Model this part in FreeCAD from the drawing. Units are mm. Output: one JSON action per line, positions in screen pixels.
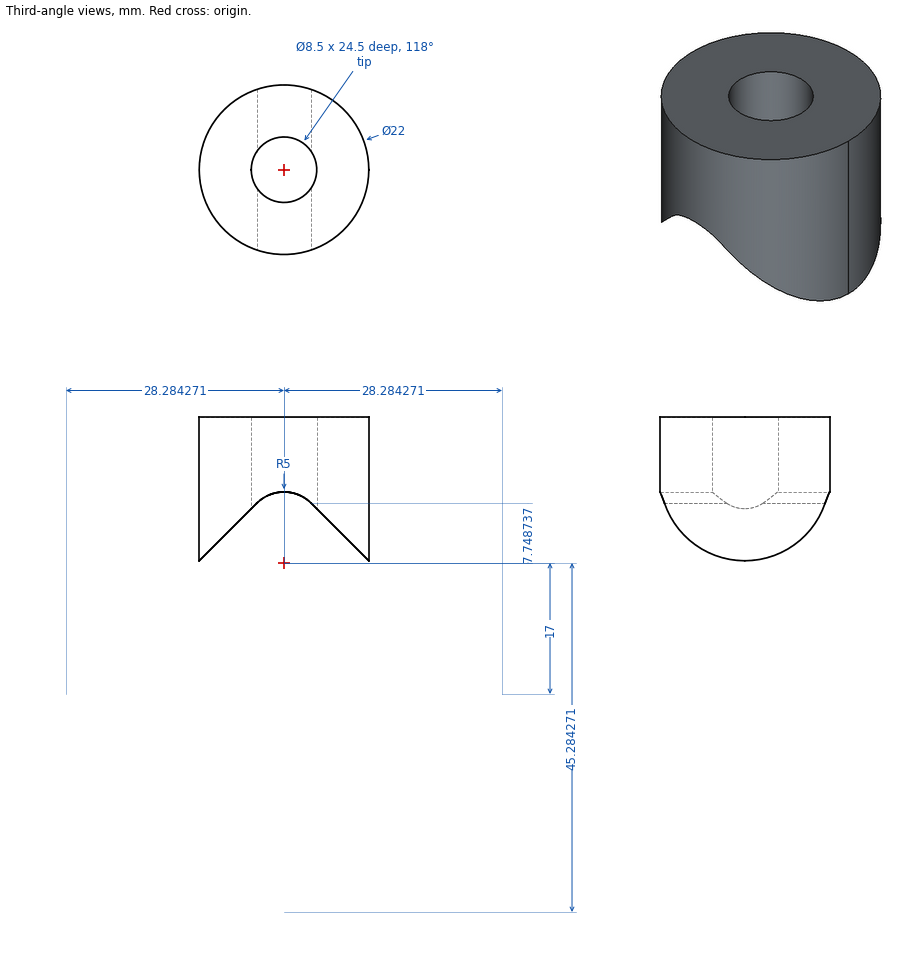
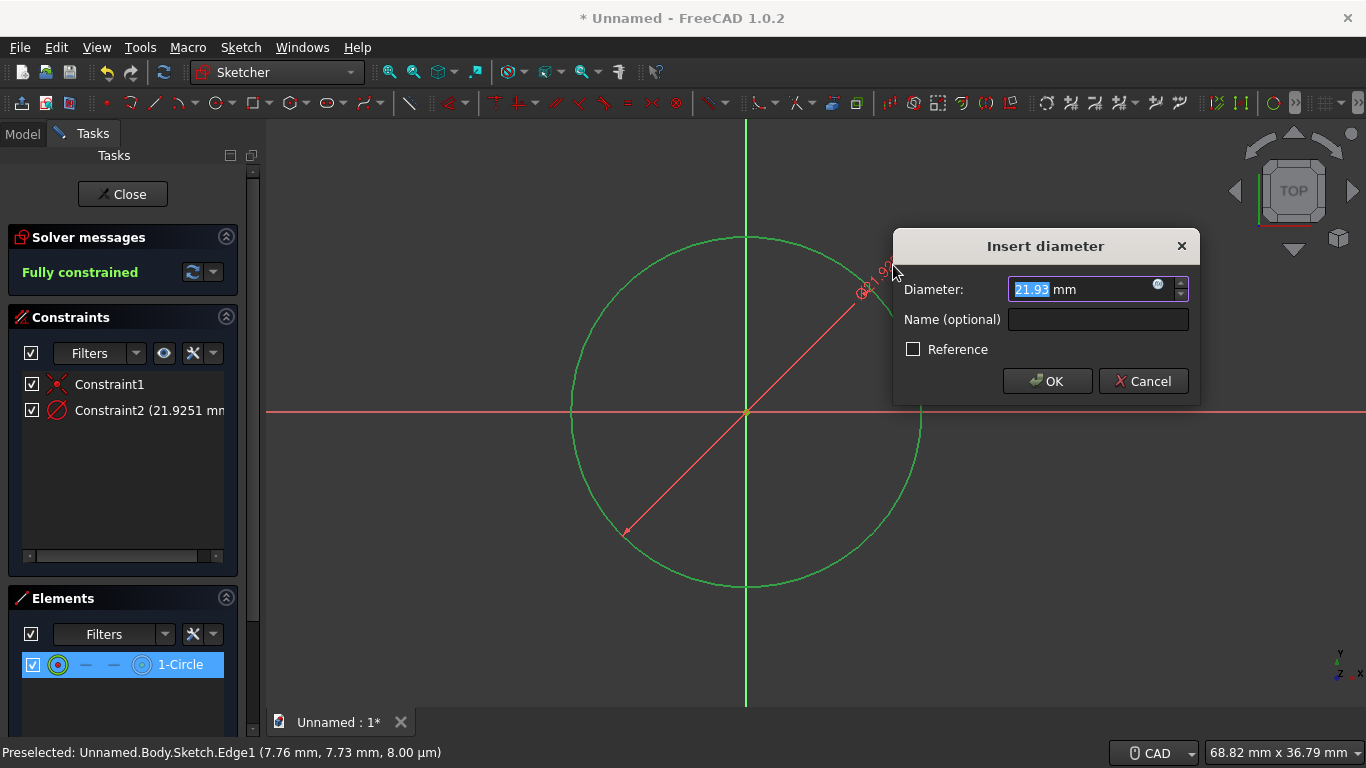
{"action": "type", "text": "22"}
{"action": "key", "text": "Return"}
{"action": "key", "text": "Escape"}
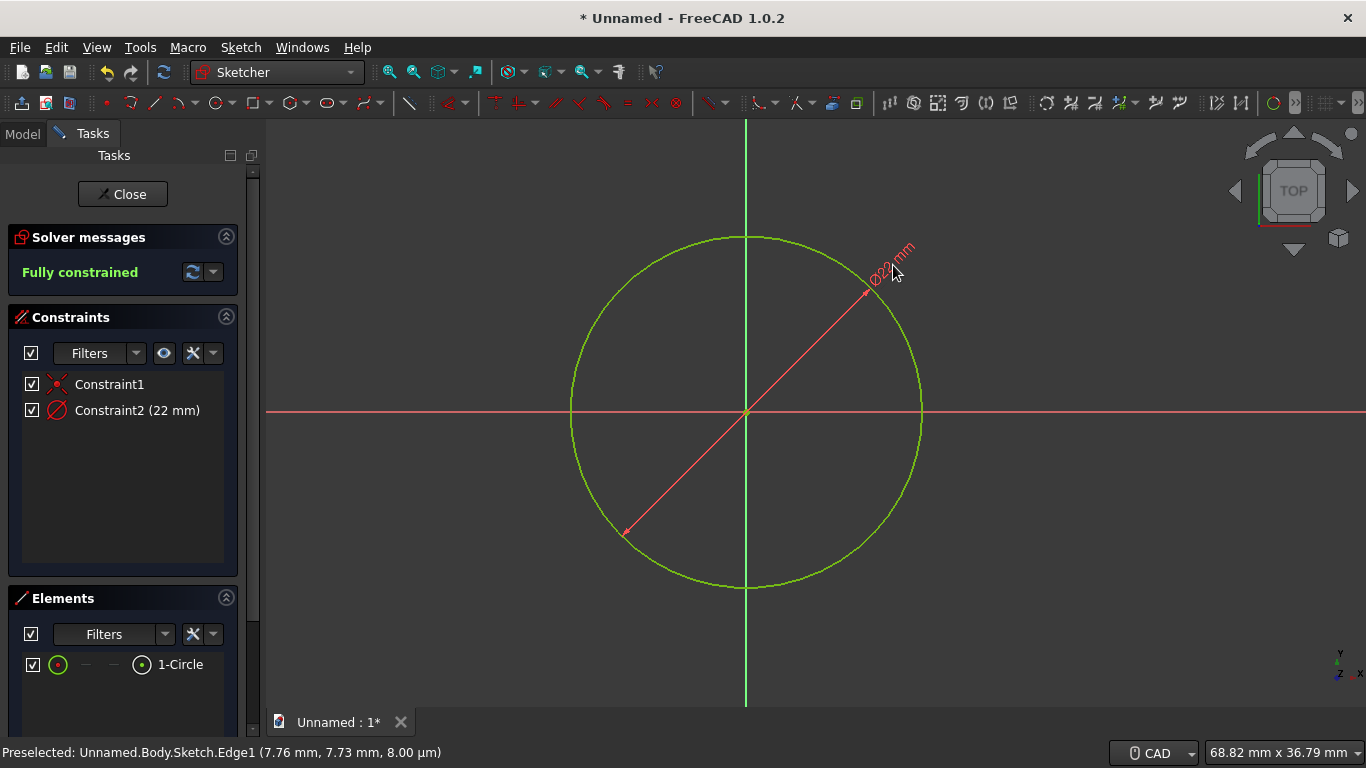
{"action": "left_click", "coordinate": [123, 194]}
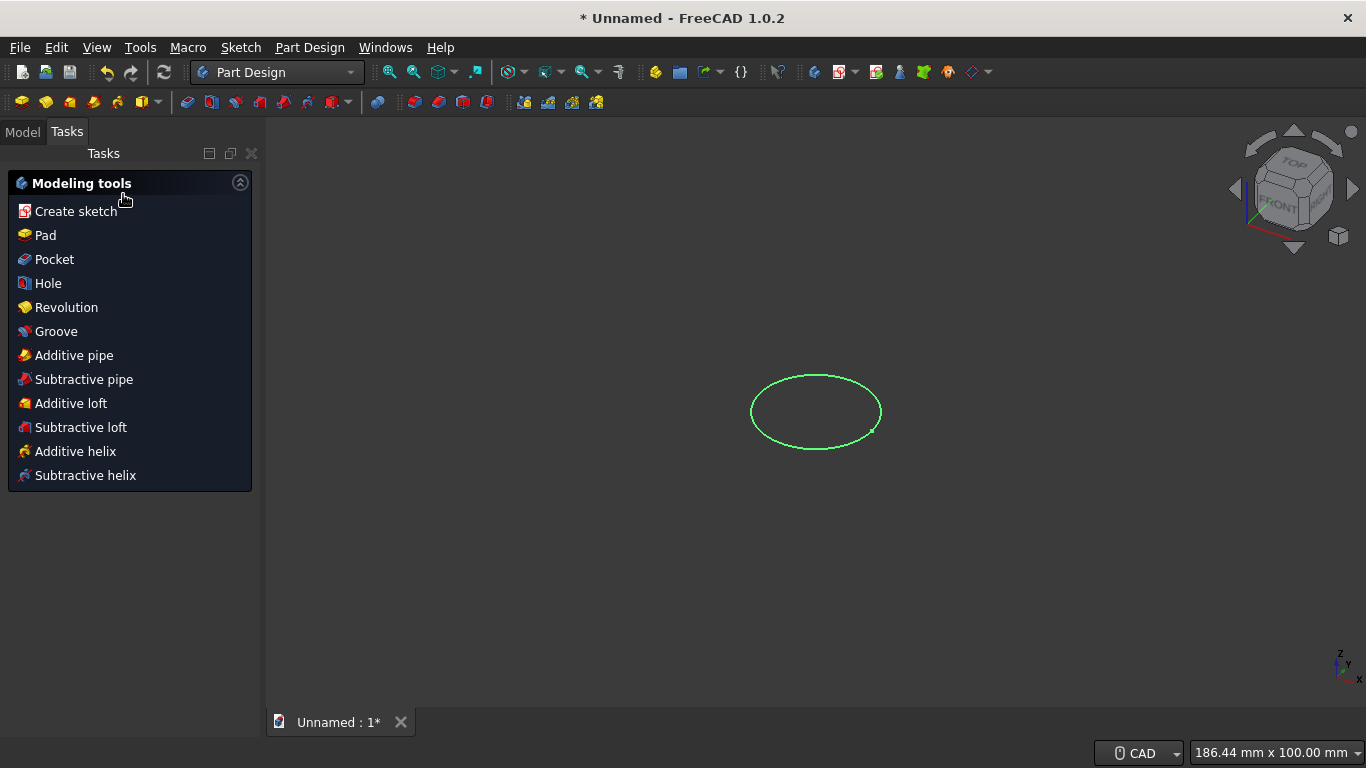
{"action": "left_click", "coordinate": [22, 102]}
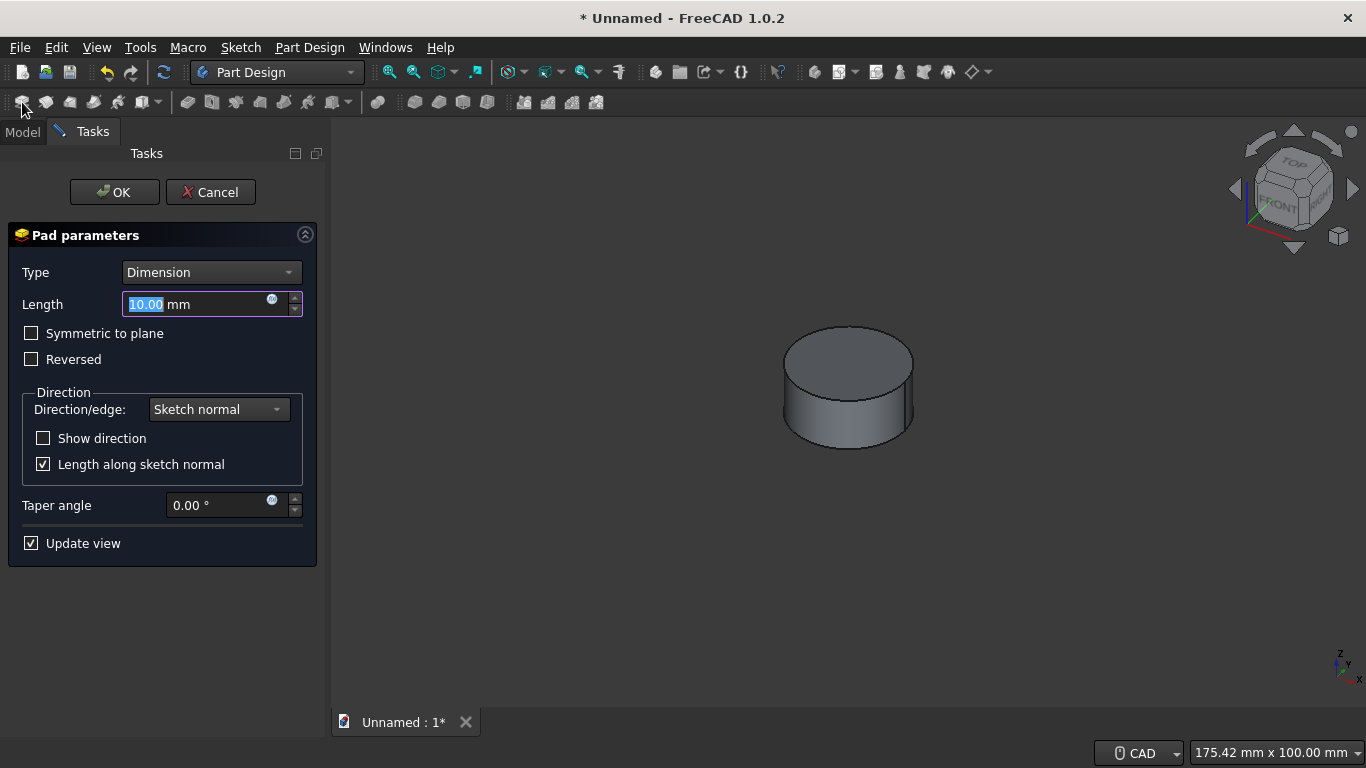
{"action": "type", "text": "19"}
{"action": "key", "text": "Tab"}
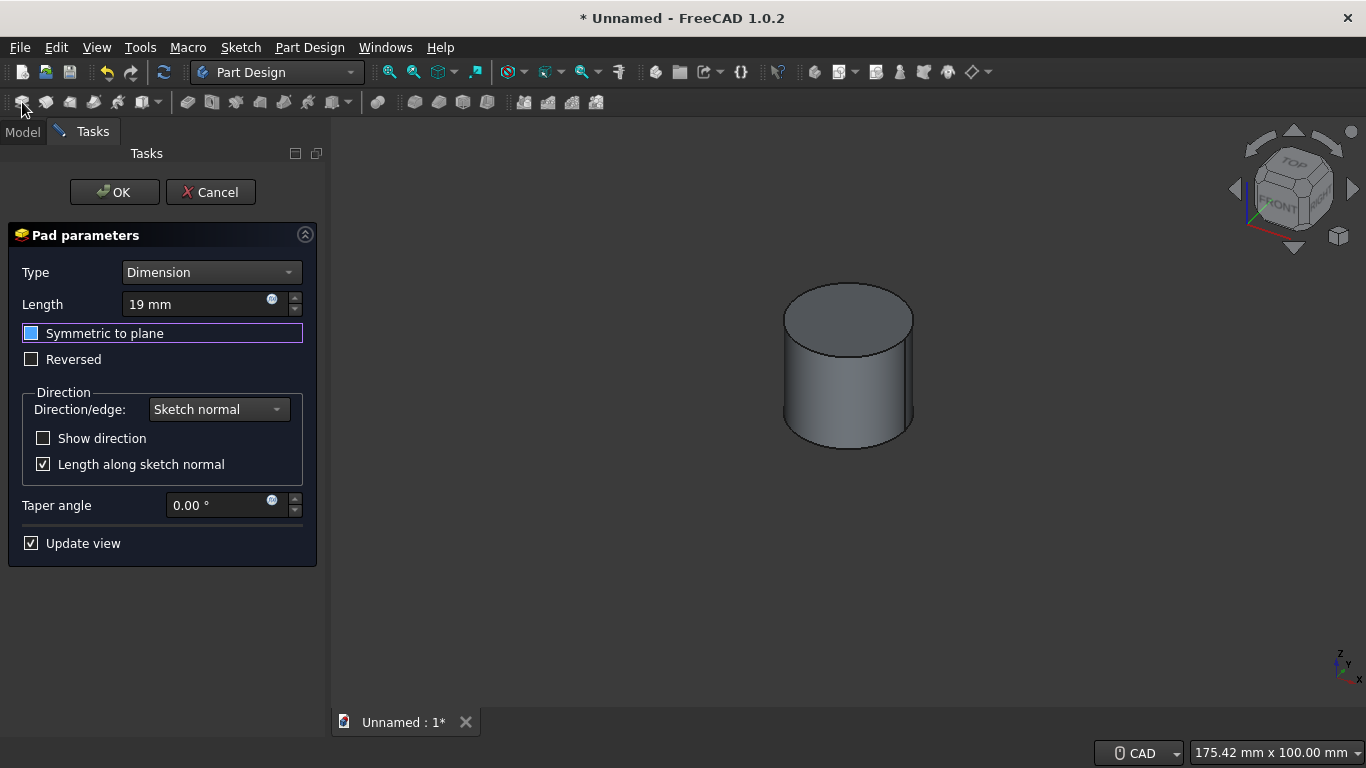
{"action": "left_click", "coordinate": [115, 192]}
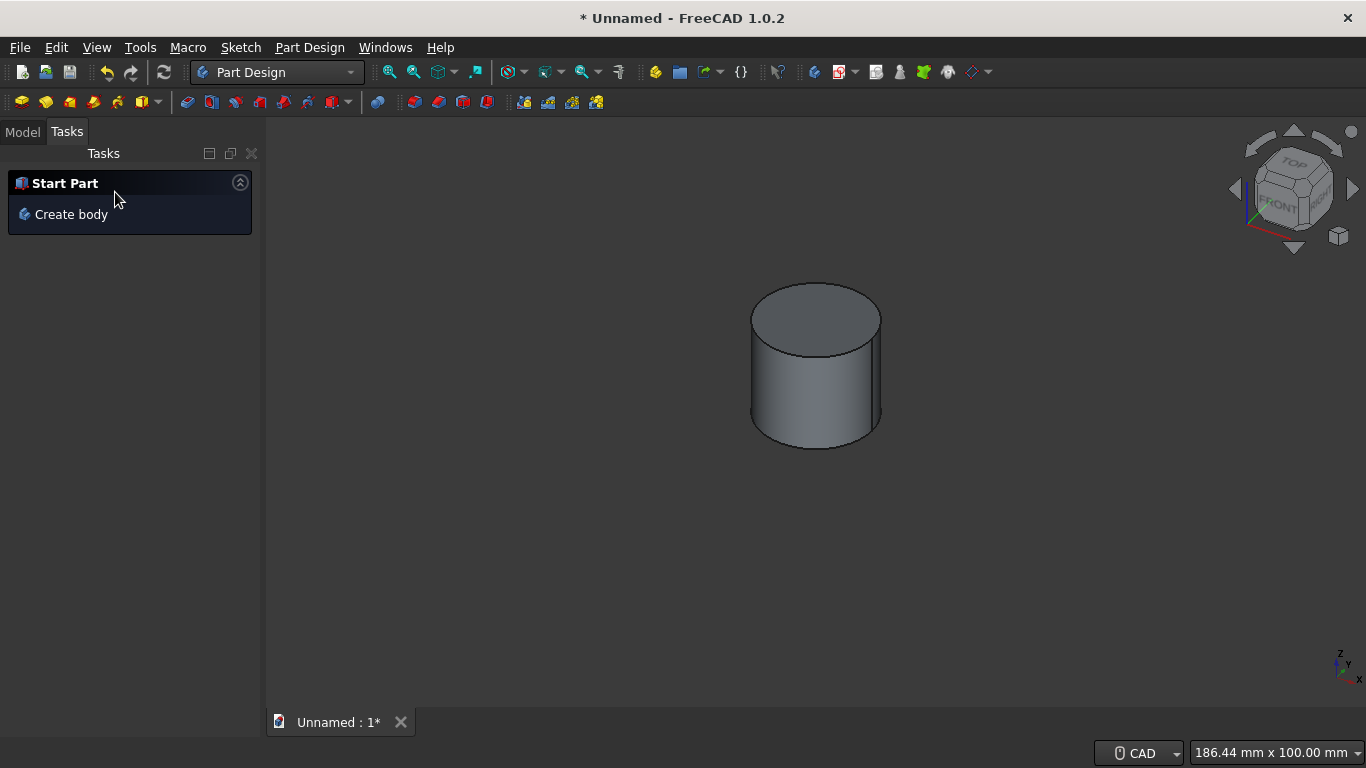
{"action": "key", "text": "v f"}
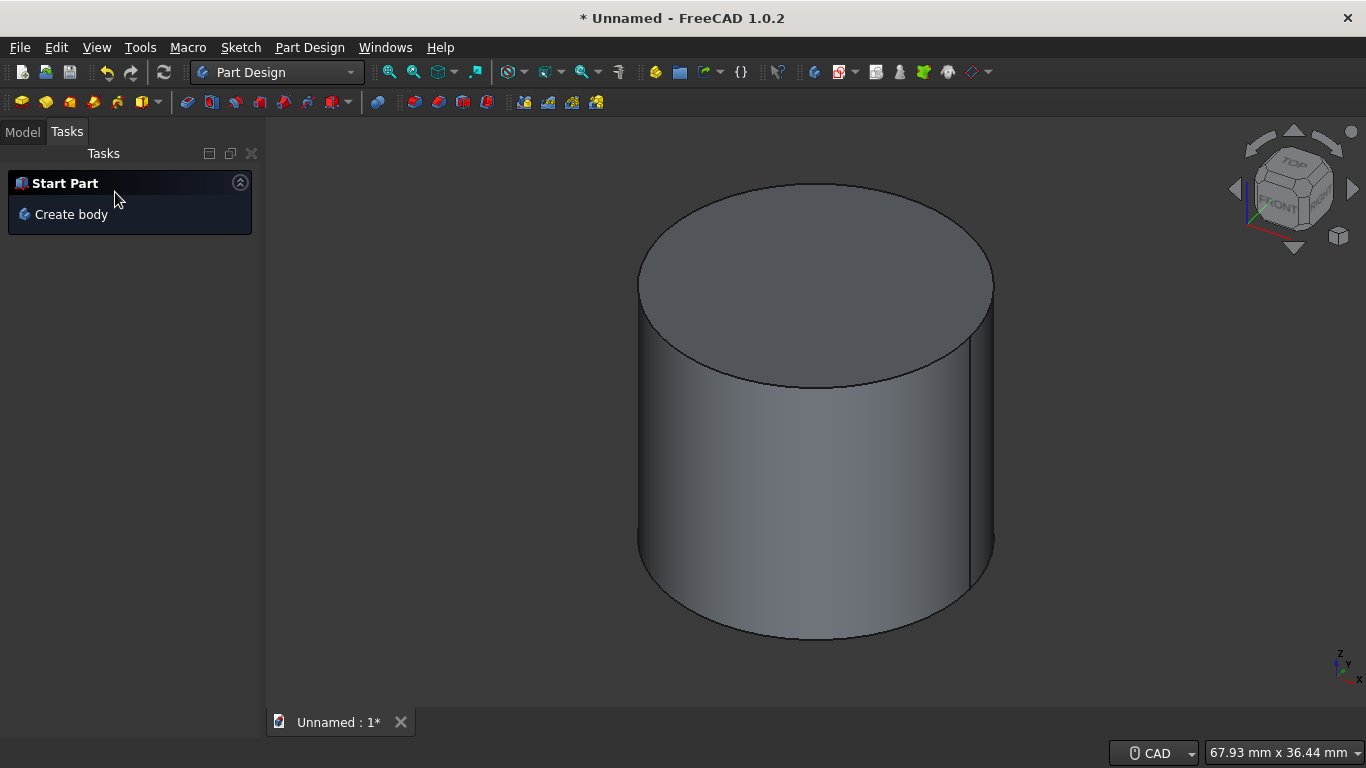
{"action": "left_click", "coordinate": [816, 285]}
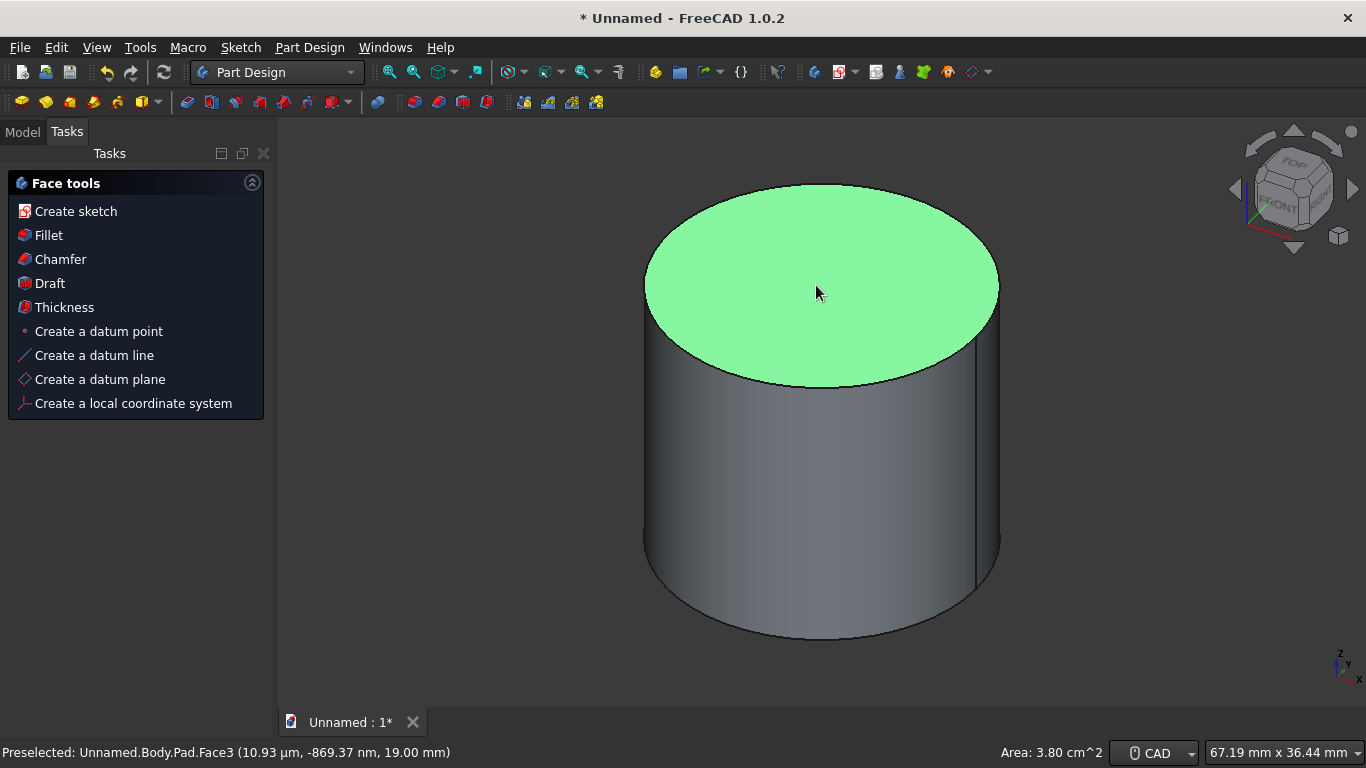
{"action": "left_click", "coordinate": [840, 72]}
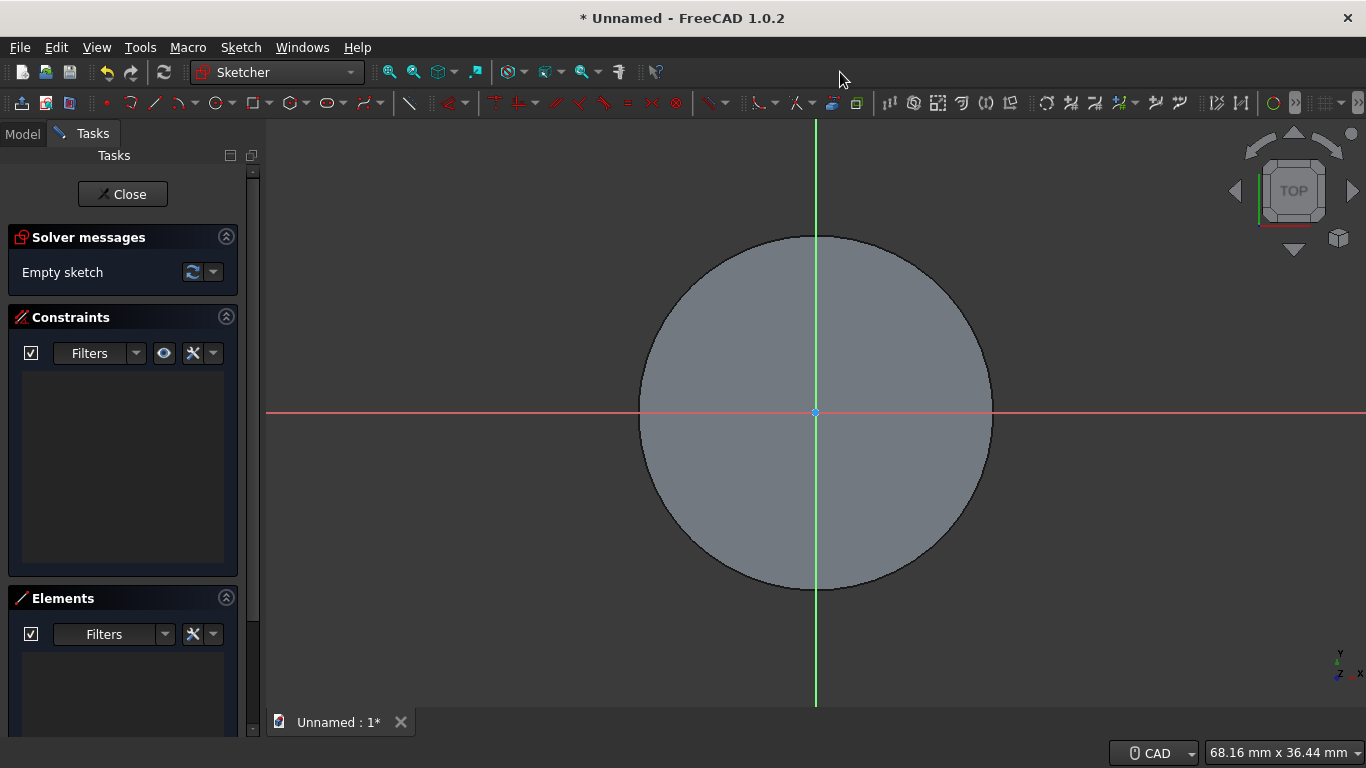
{"action": "scroll", "coordinate": [856, 413], "scroll_direction": "up", "scroll_amount": 5}